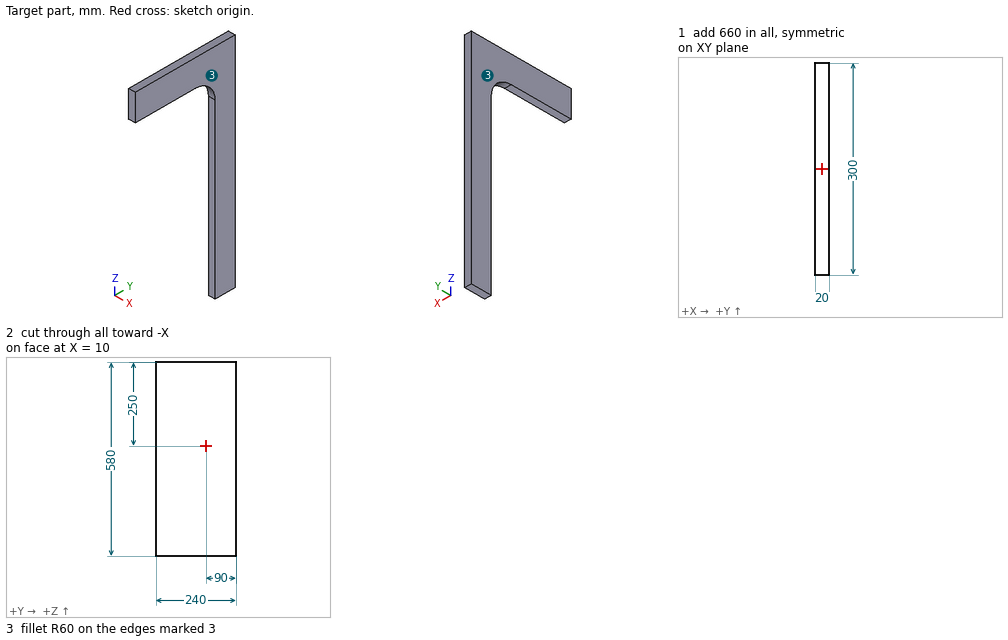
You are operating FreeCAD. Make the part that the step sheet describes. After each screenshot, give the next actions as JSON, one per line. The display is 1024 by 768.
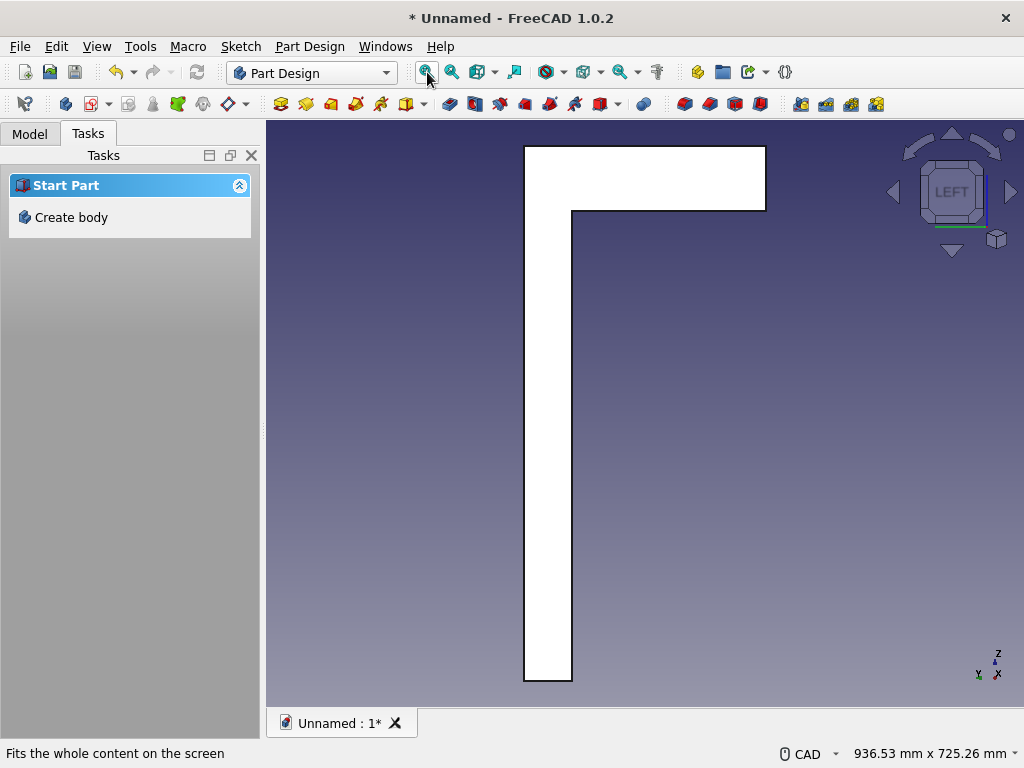
{"action": "key", "text": "v 3"}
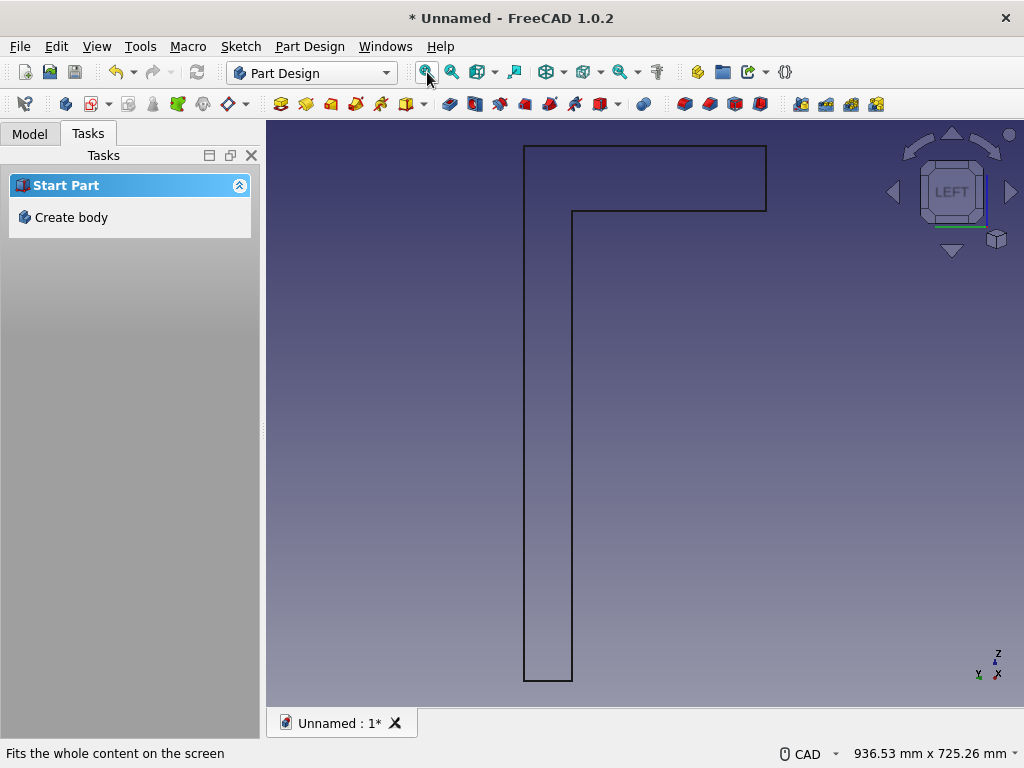
{"action": "key", "text": "0"}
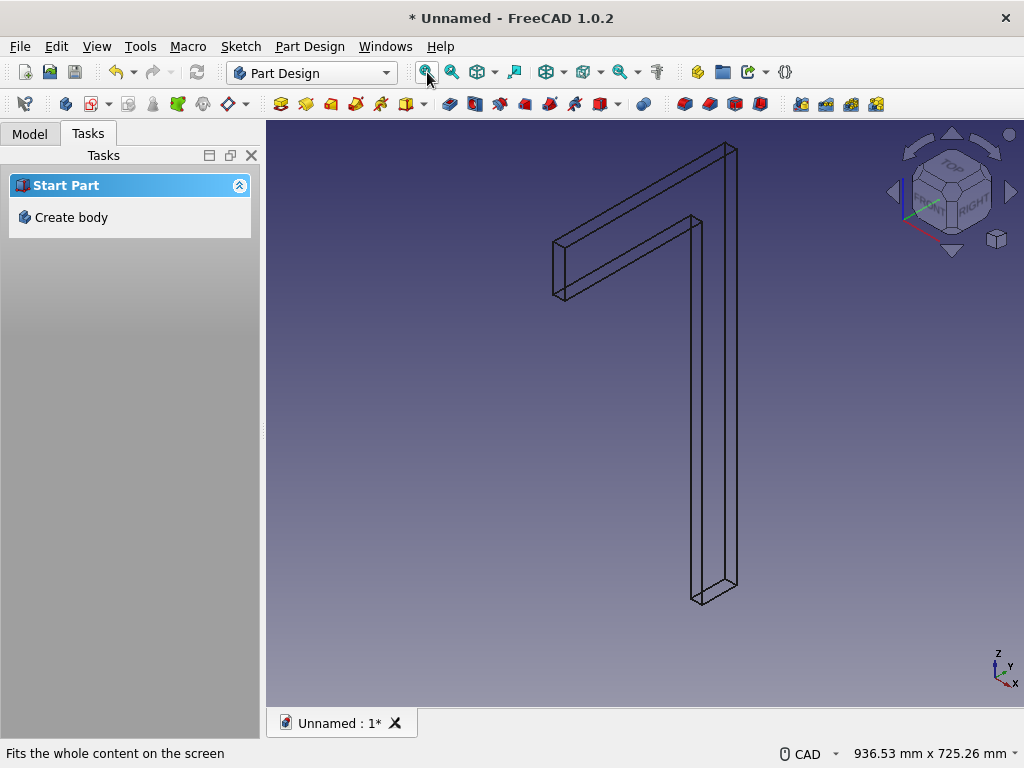
{"action": "left_click", "coordinate": [695, 217]}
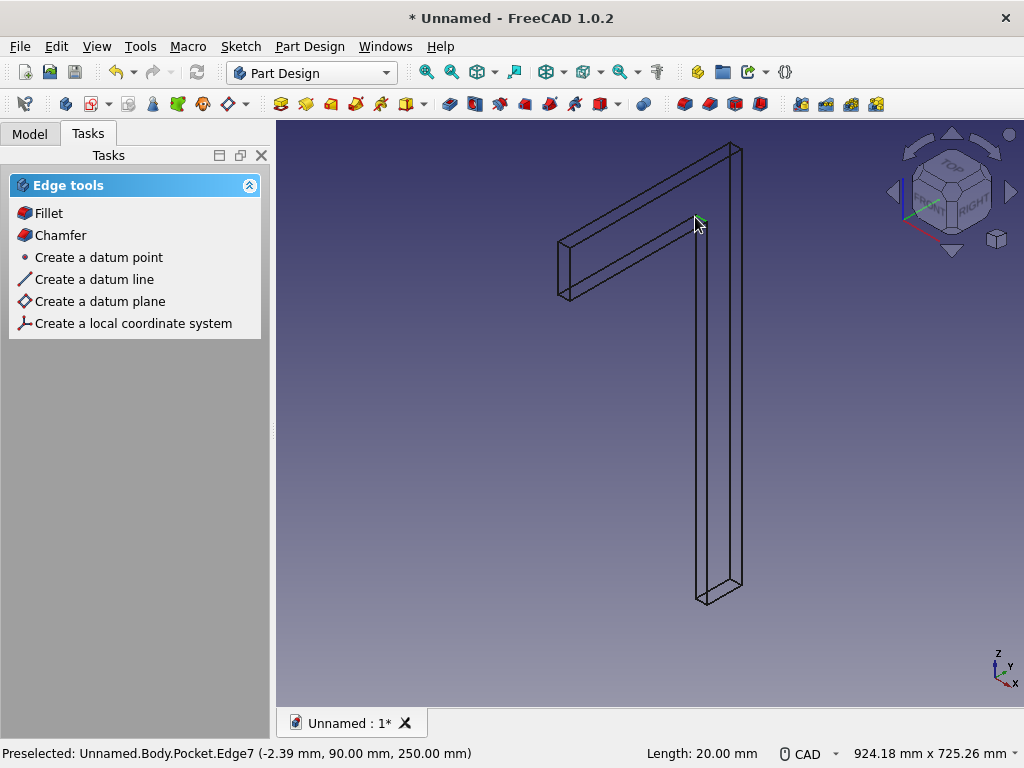
{"action": "key", "text": "v 1"}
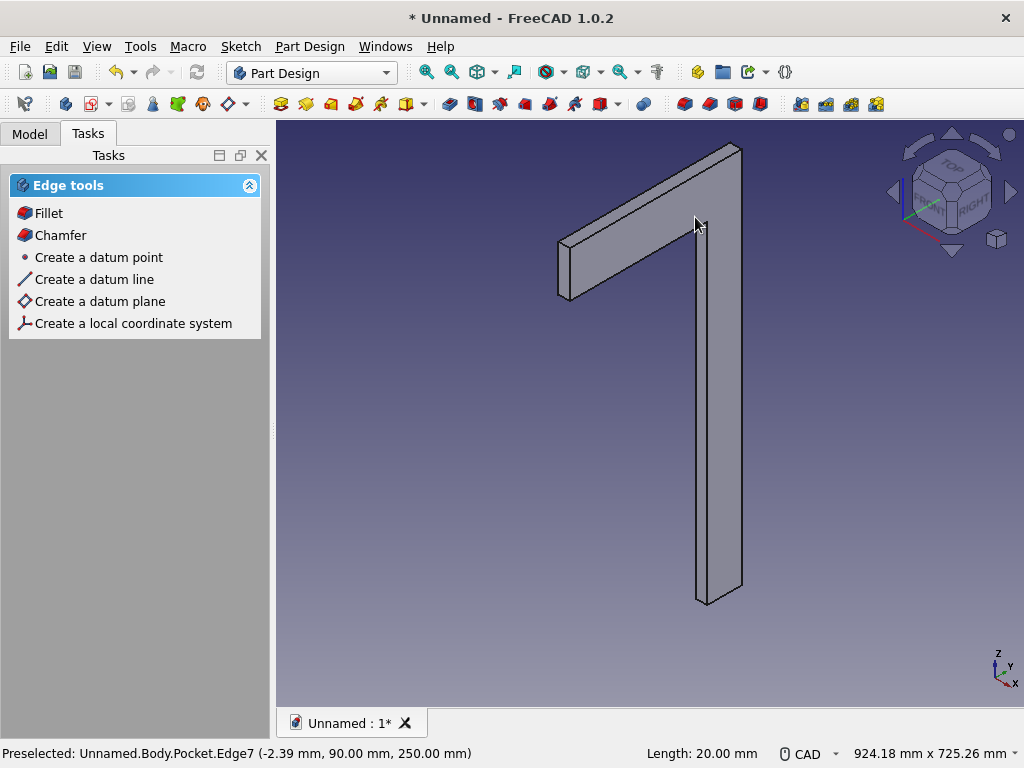
{"action": "left_click", "coordinate": [685, 104]}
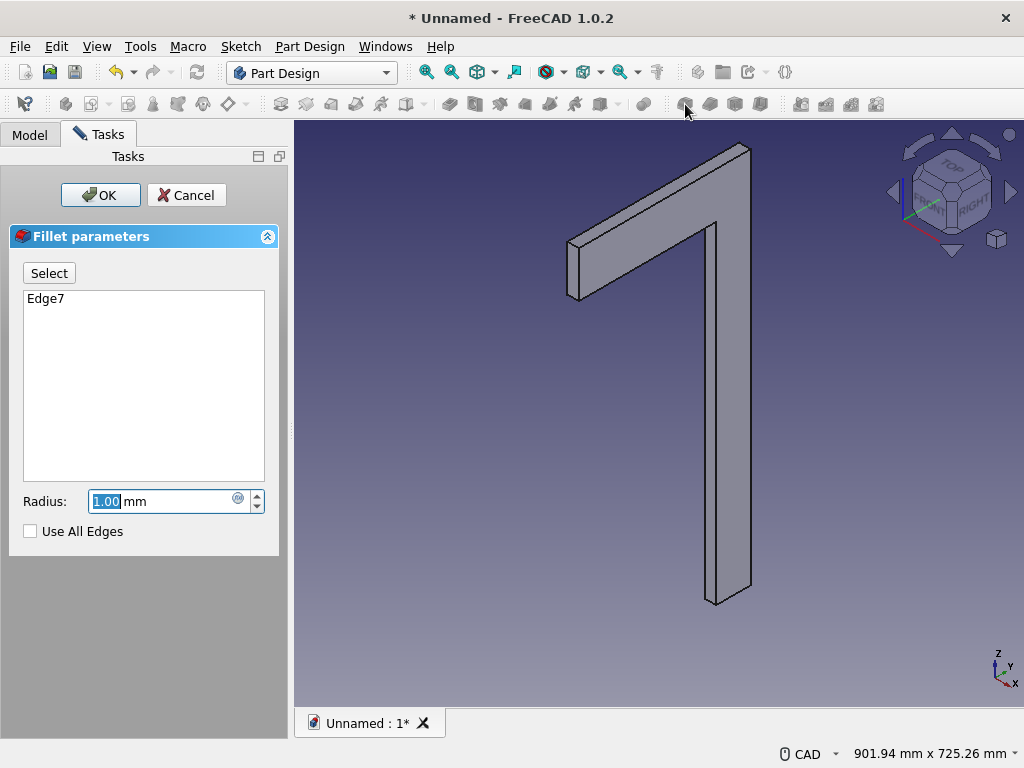
{"action": "type", "text": "60"}
{"action": "key", "text": "Tab"}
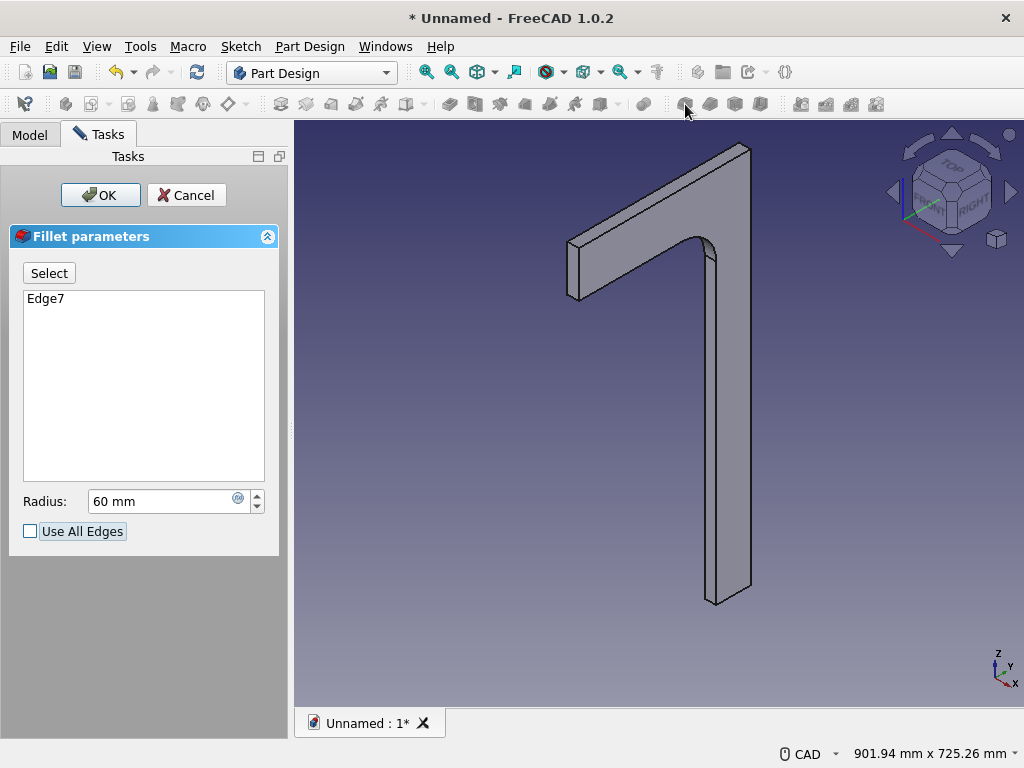
{"action": "left_click", "coordinate": [101, 195]}